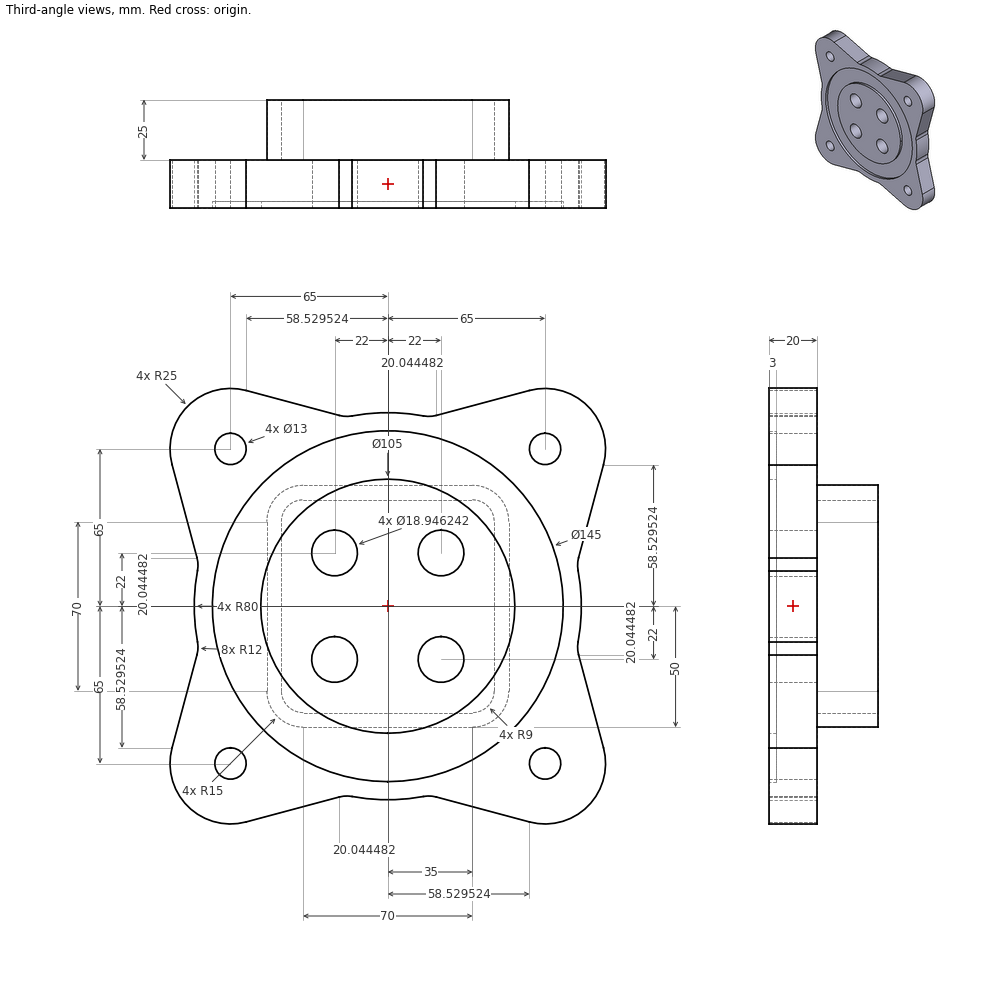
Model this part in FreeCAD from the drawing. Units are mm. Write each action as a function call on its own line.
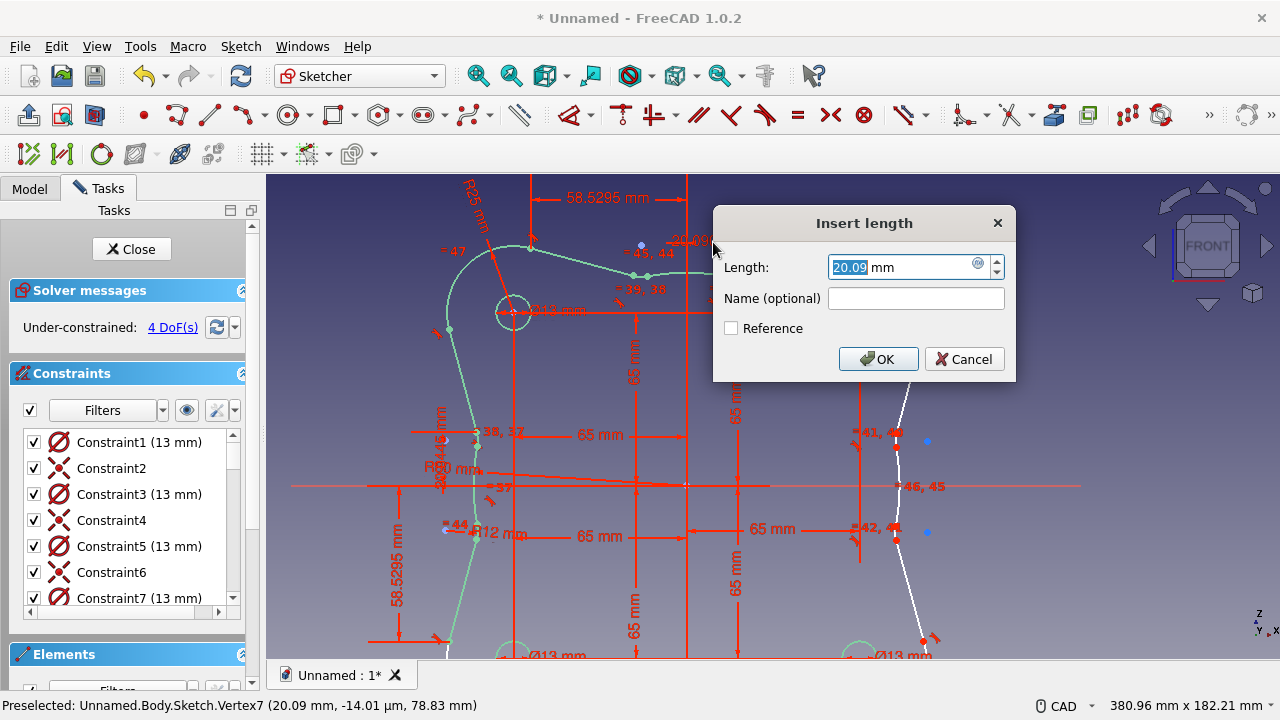
text(20.044482)
key(Return)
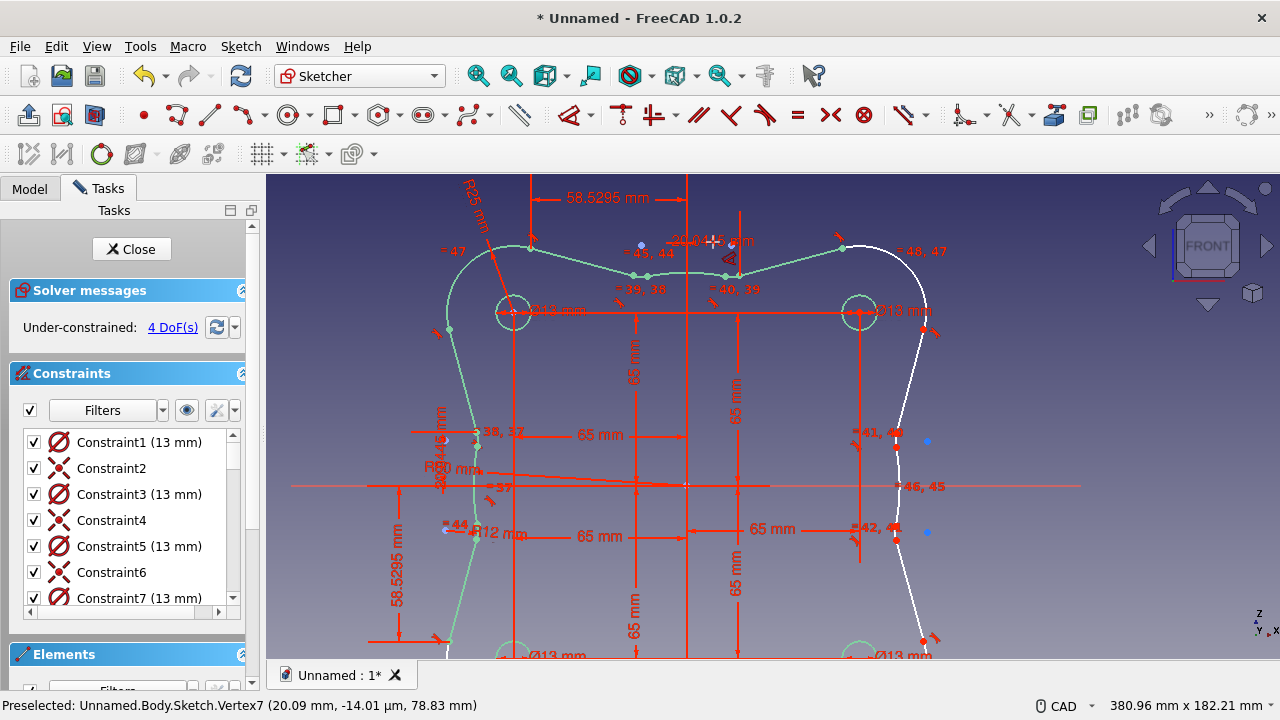
click(924, 330)
click(958, 408)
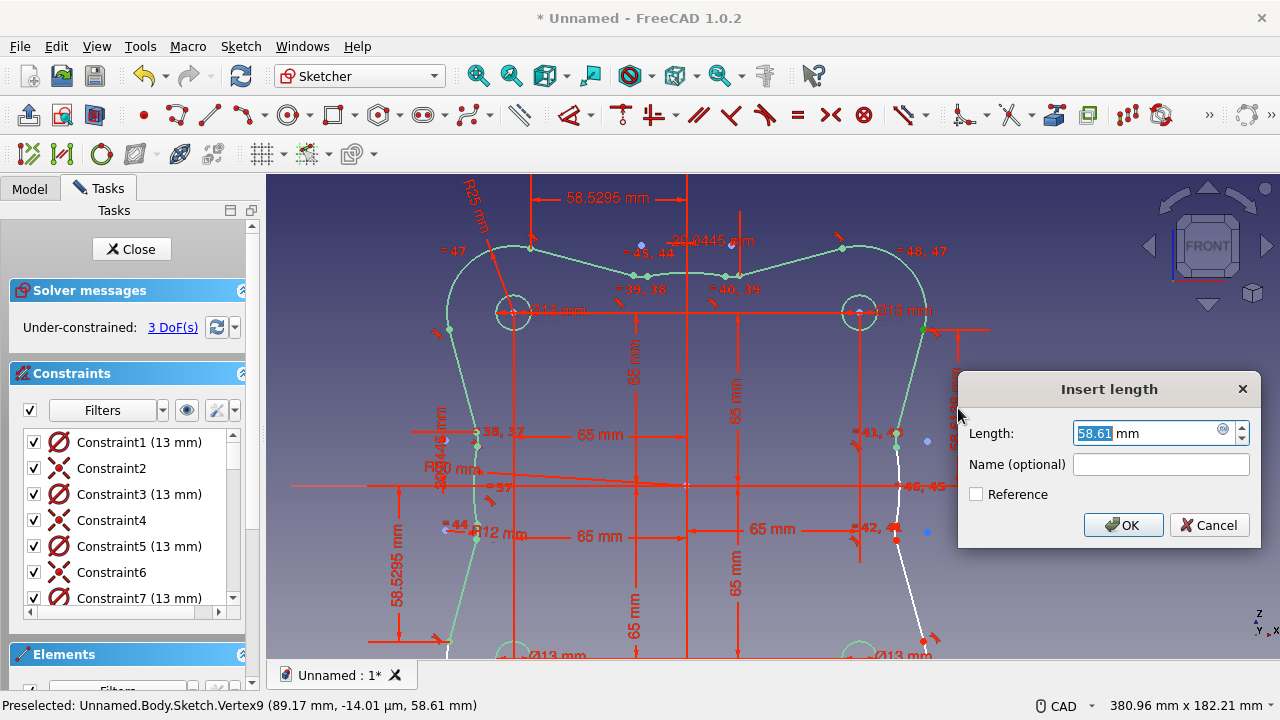
text(58.529524)
key(Return)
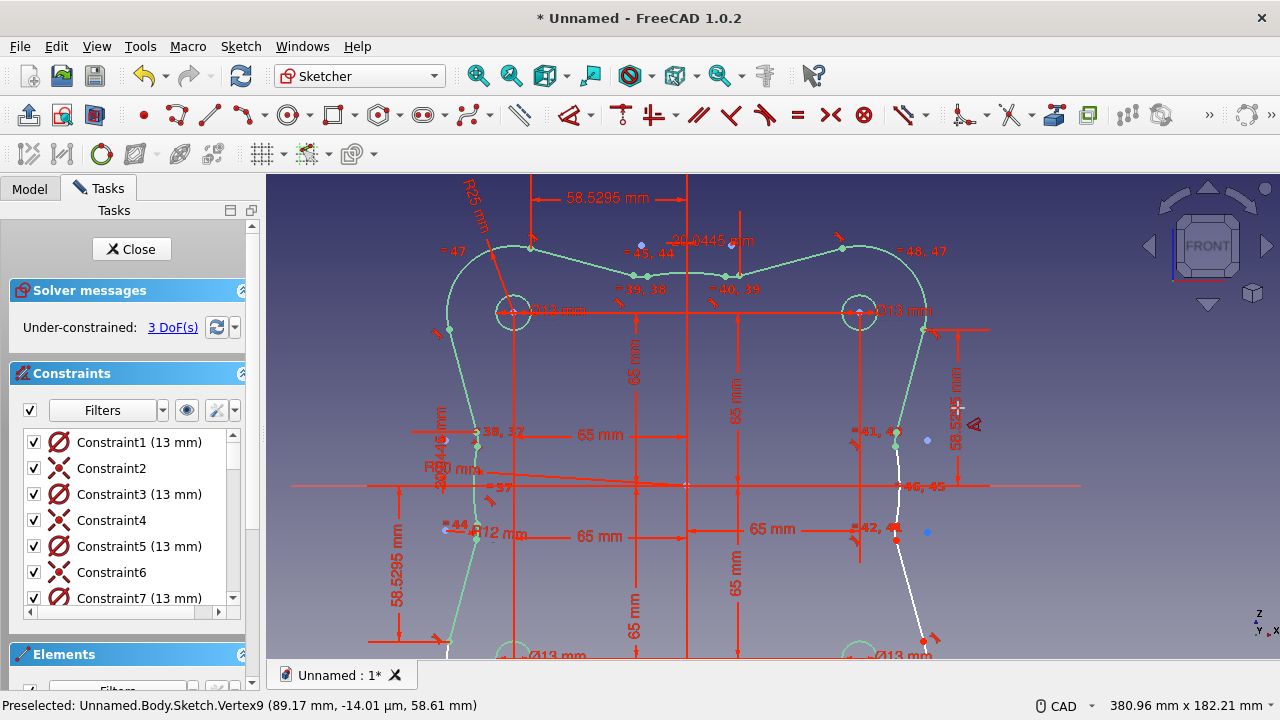
click(896, 541)
click(930, 513)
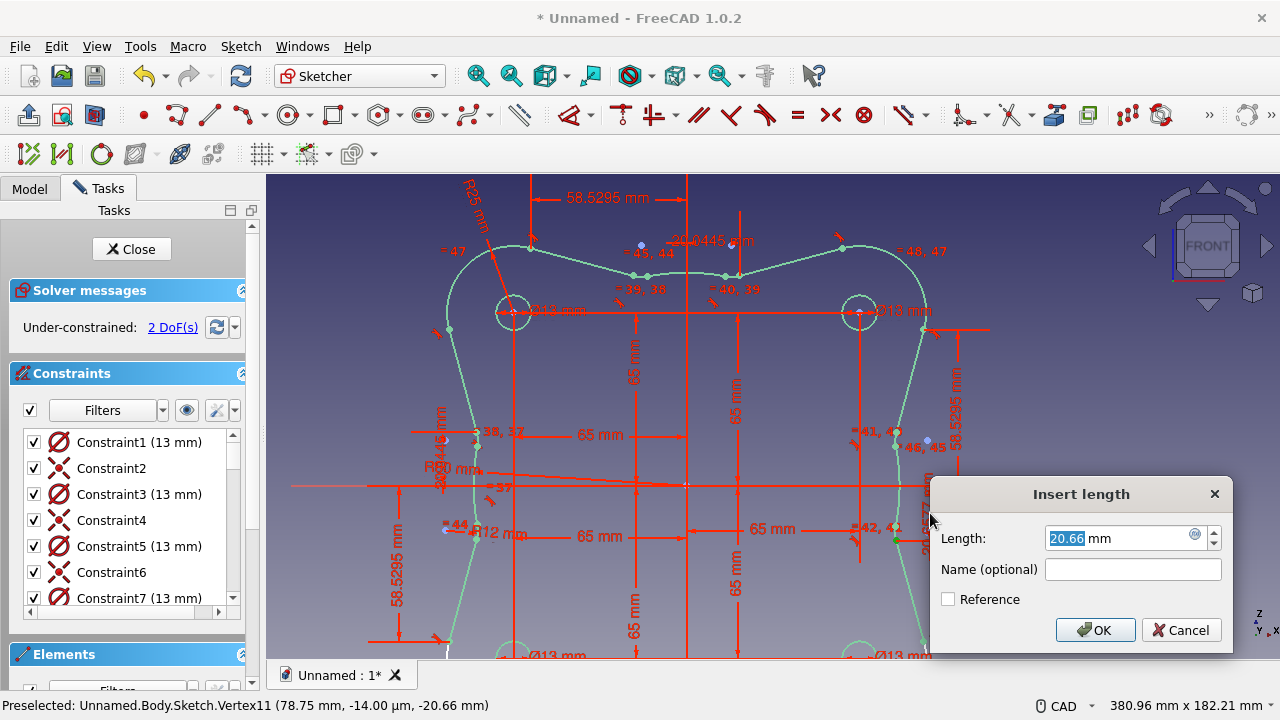
text(20.044482)
key(Return)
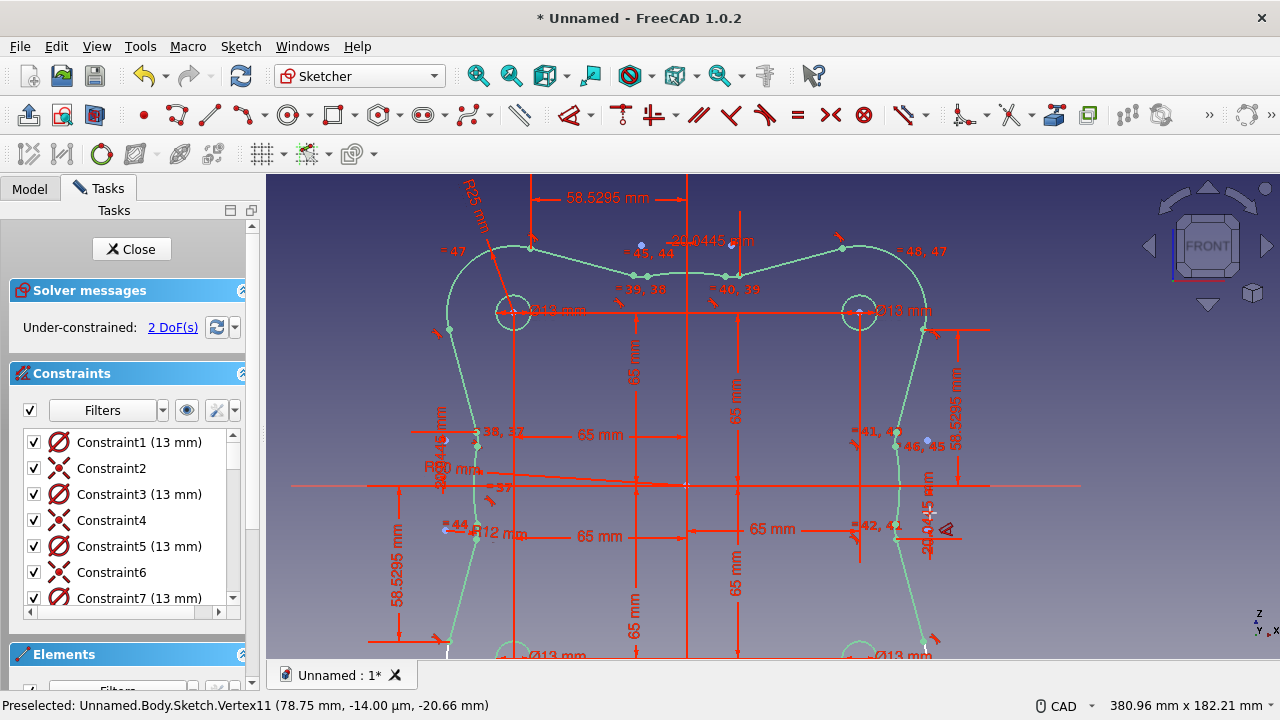
scroll(741, 276, down, 2)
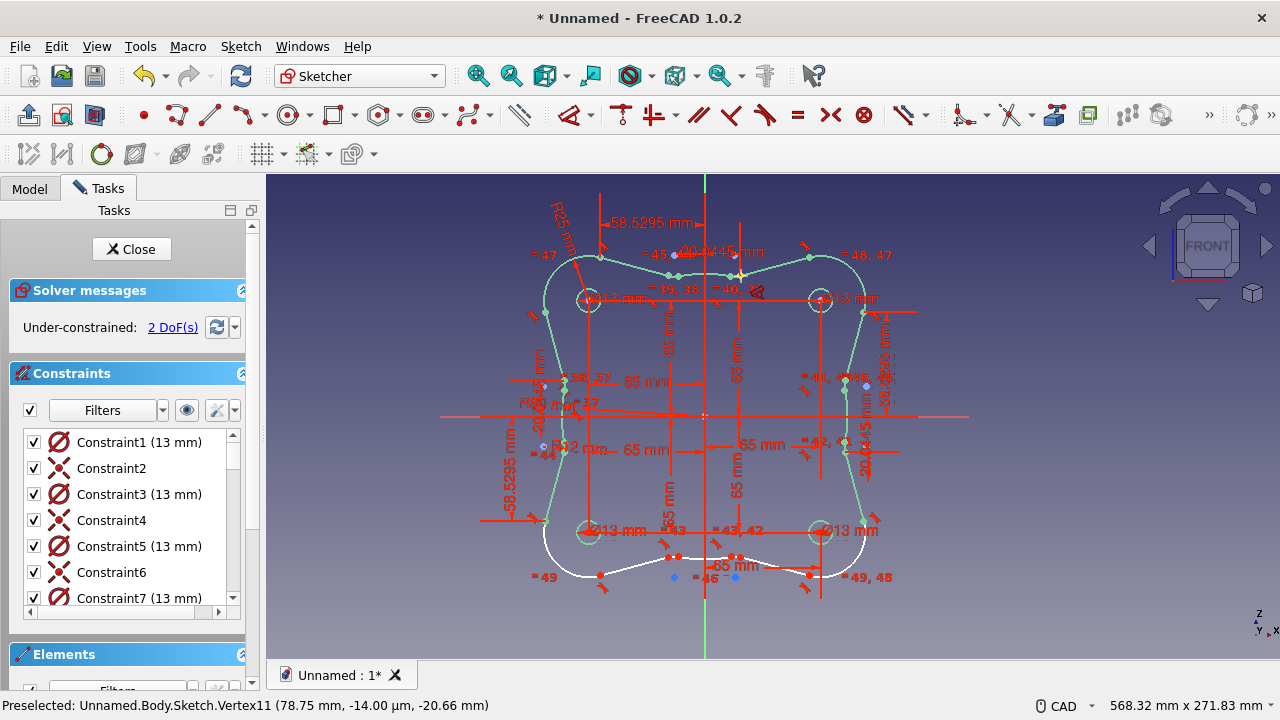
click(809, 576)
click(757, 610)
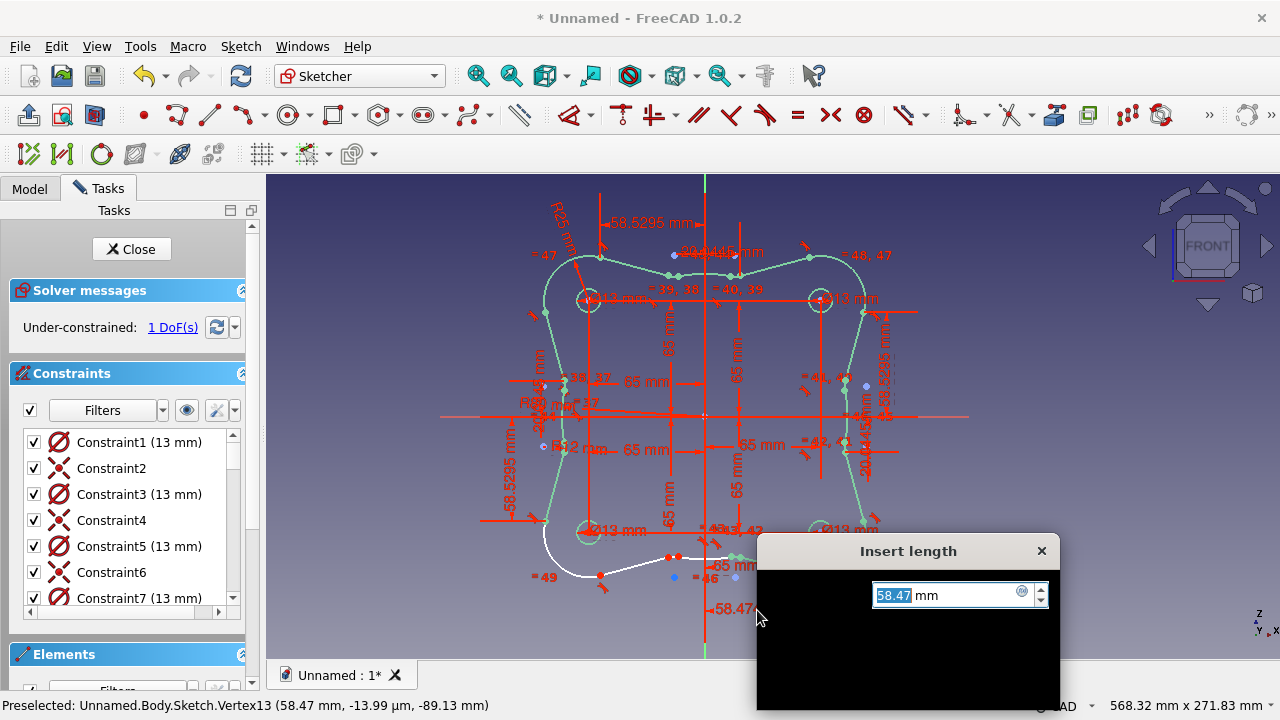
text(58.529524)
key(Return)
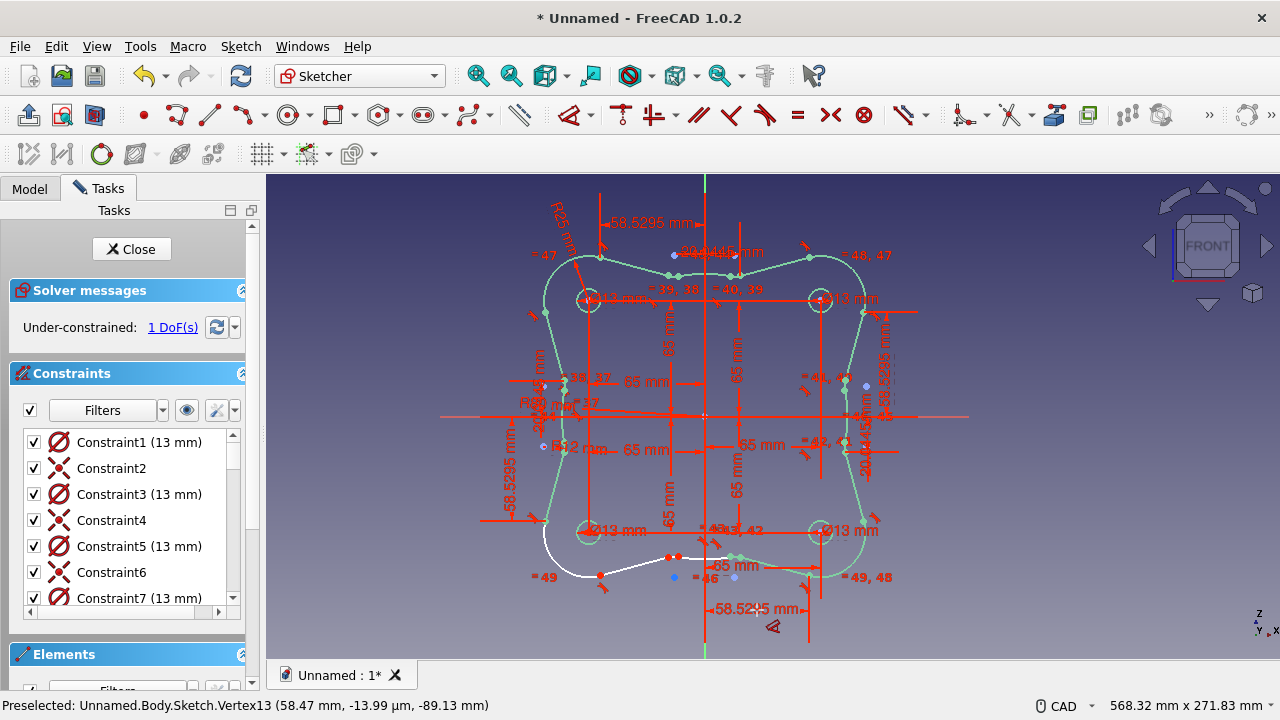
scroll(669, 557, up, 2)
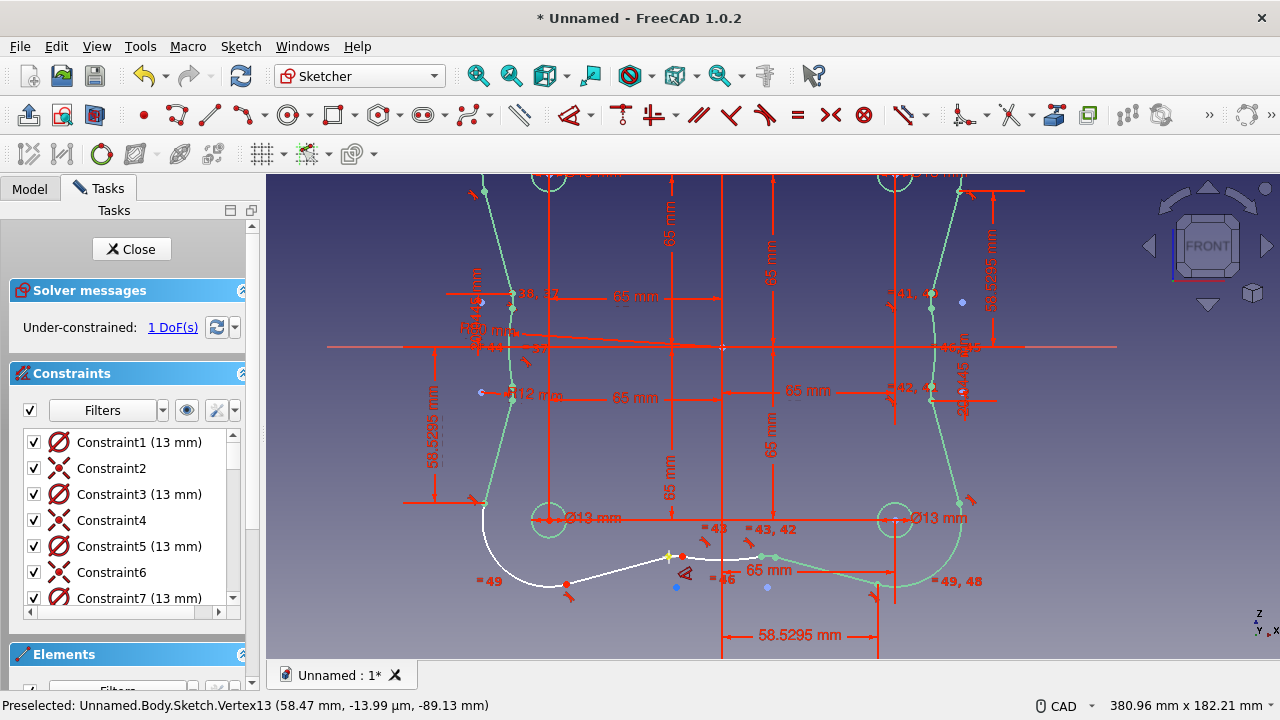
click(668, 557)
click(695, 591)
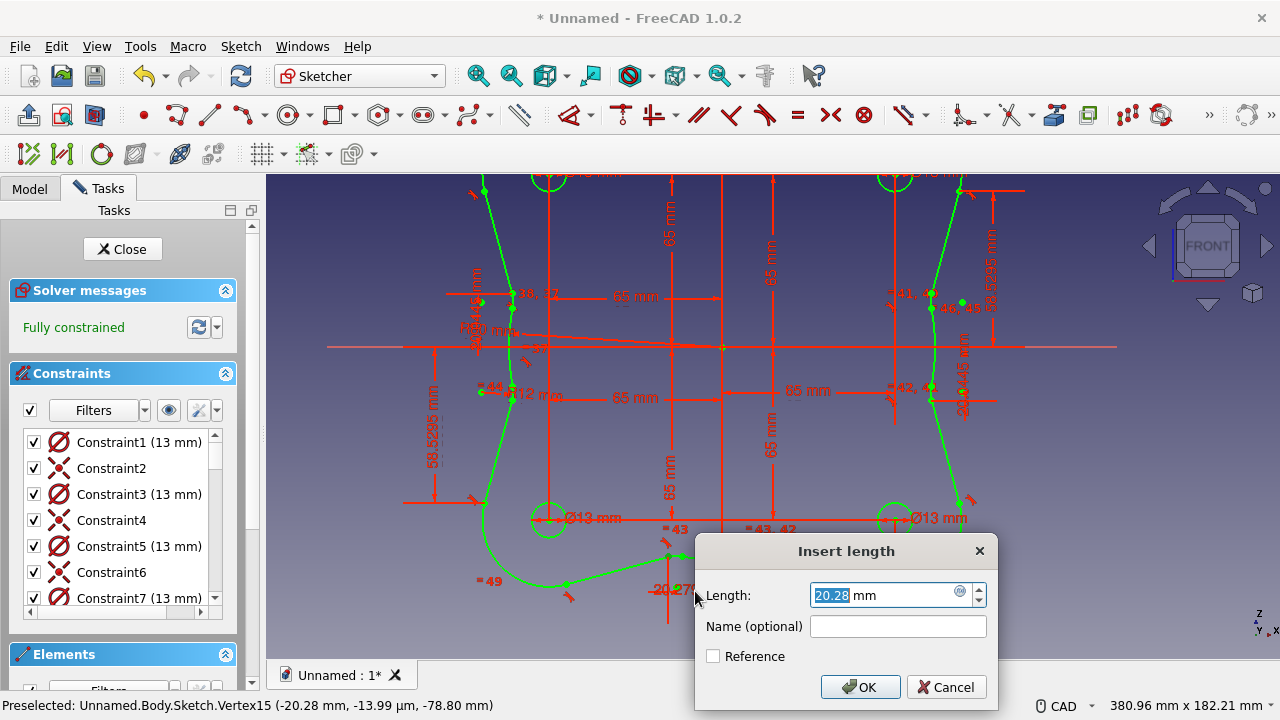
text(20.044482)
key(Return)
key(Escape)